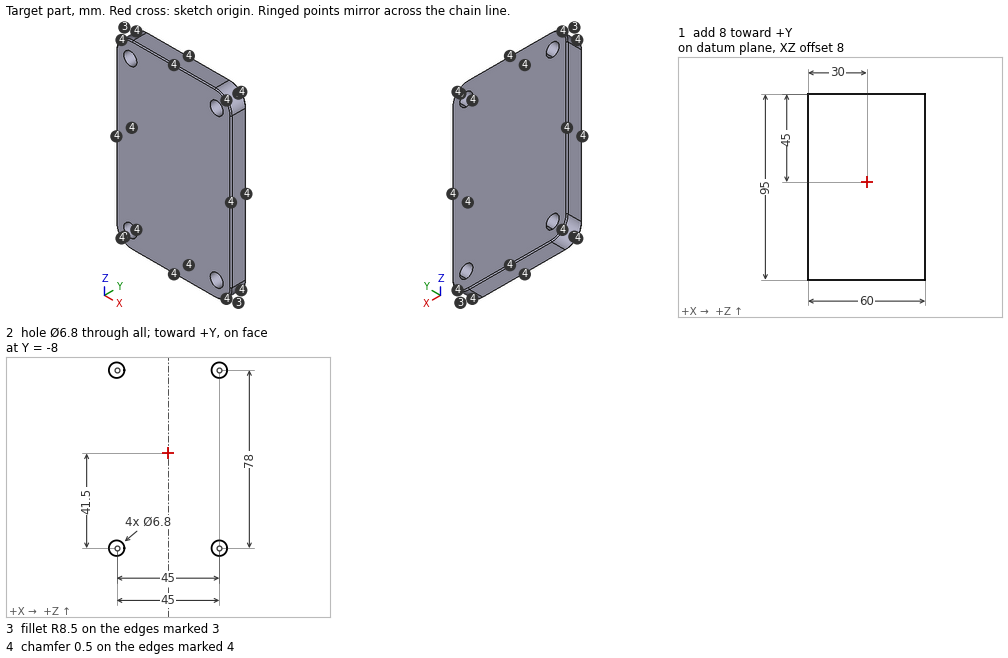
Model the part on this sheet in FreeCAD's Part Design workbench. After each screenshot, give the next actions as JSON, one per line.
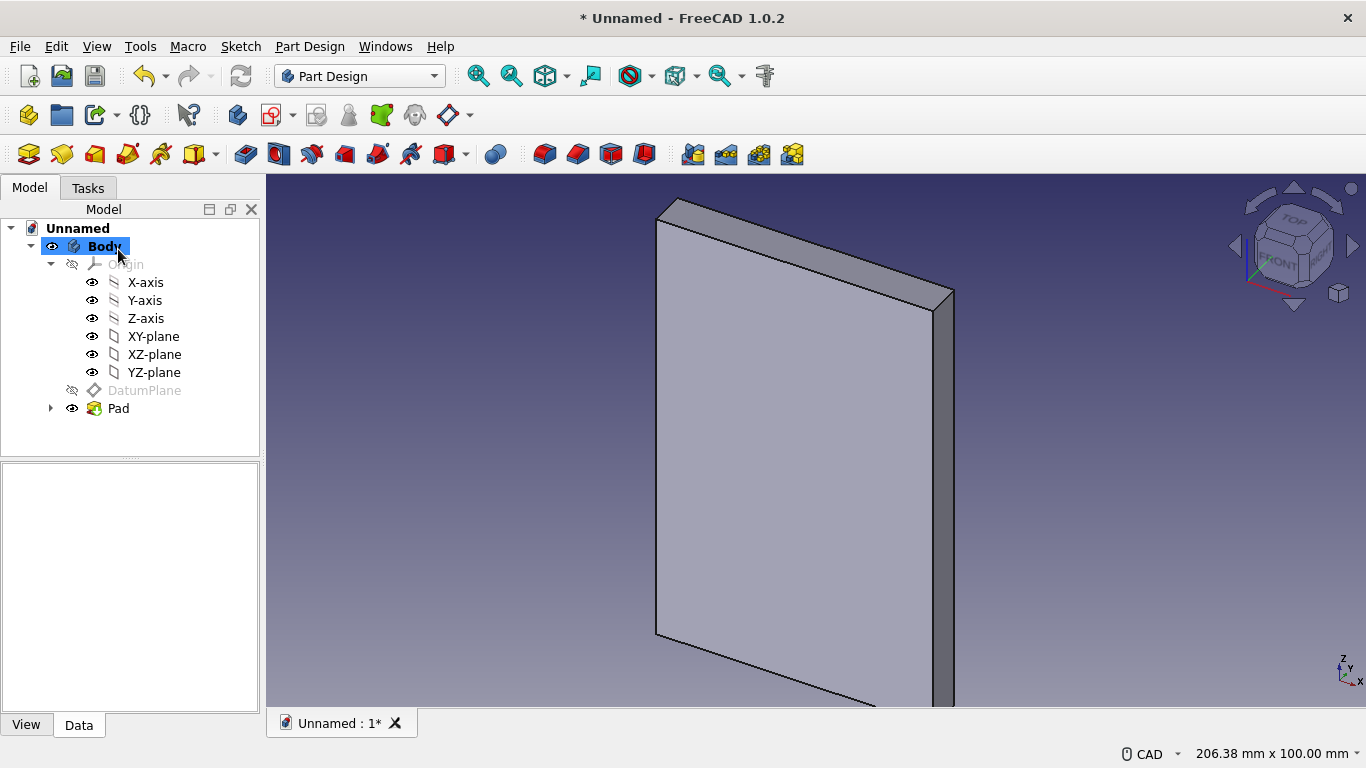
{"action": "left_click", "coordinate": [479, 76]}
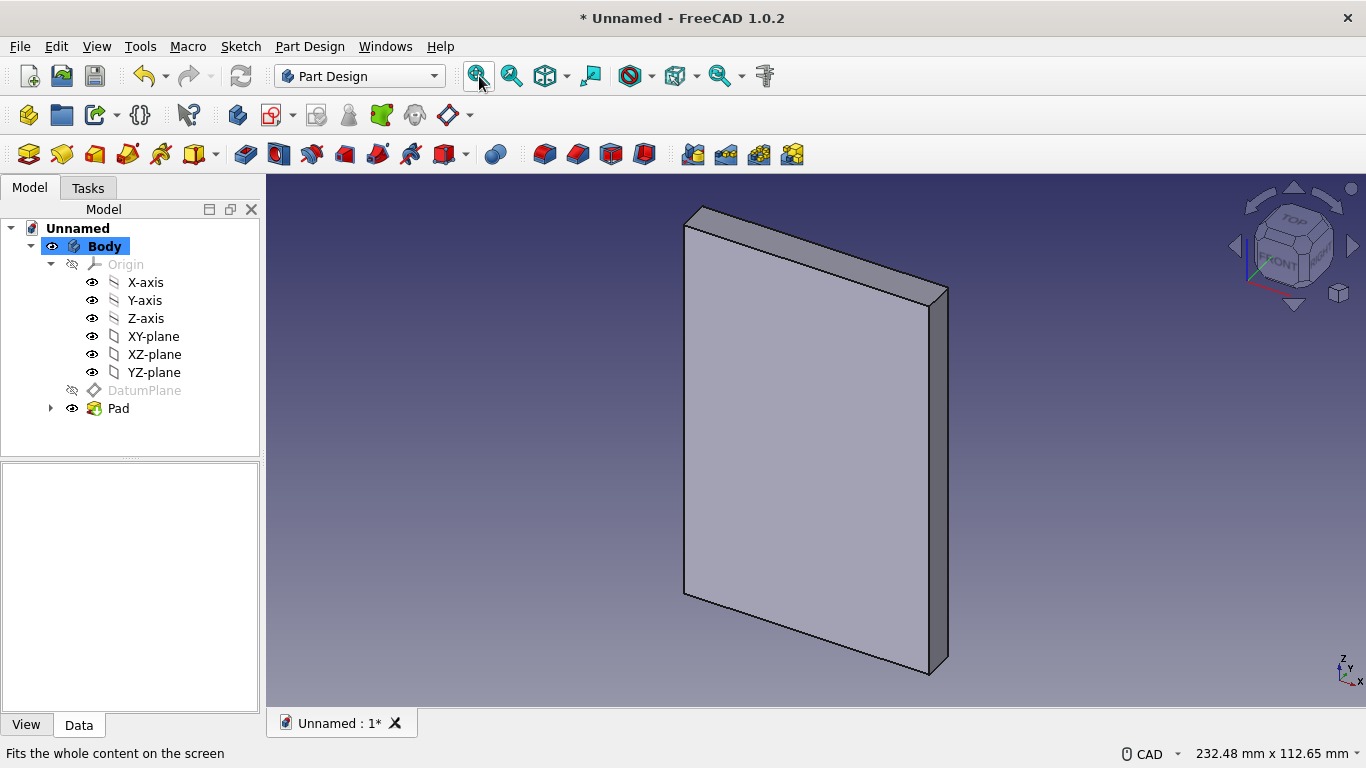
{"action": "left_click", "coordinate": [807, 396]}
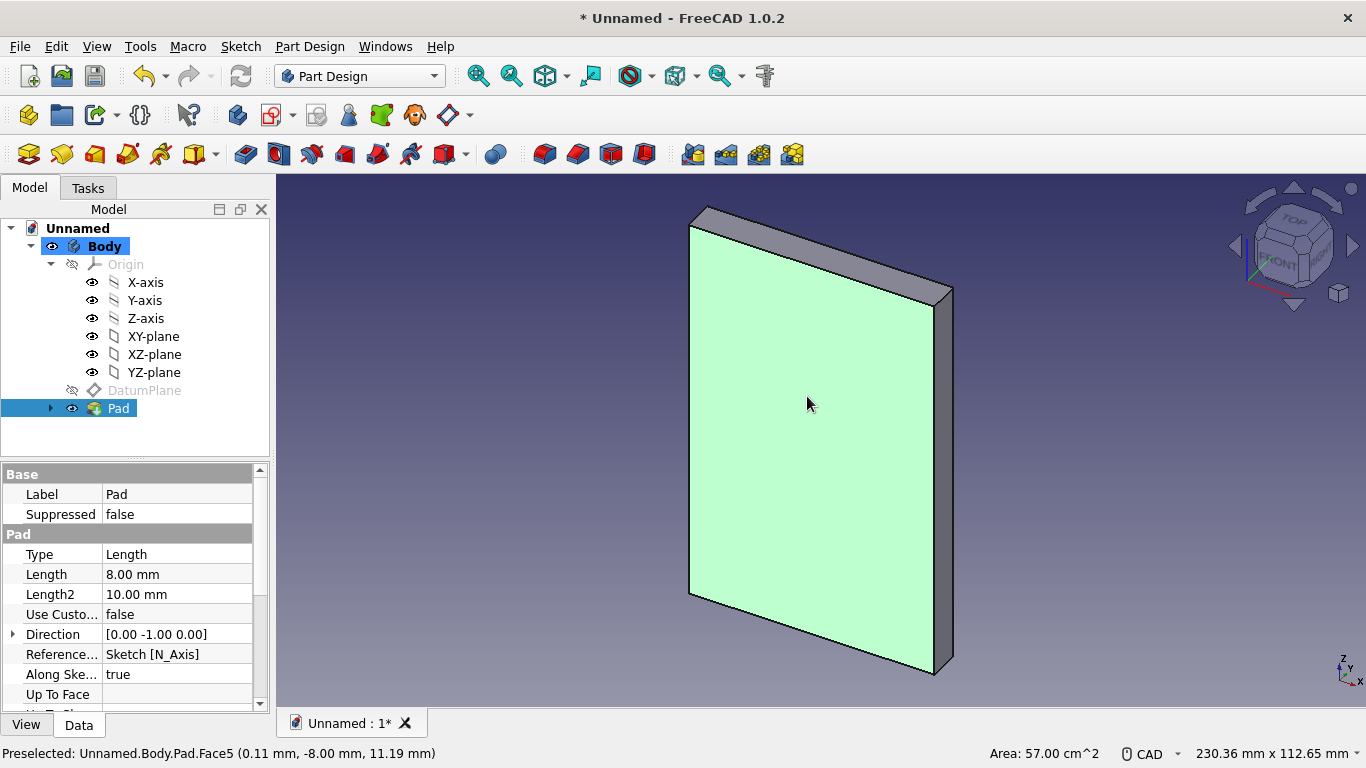
{"action": "left_click", "coordinate": [270, 116]}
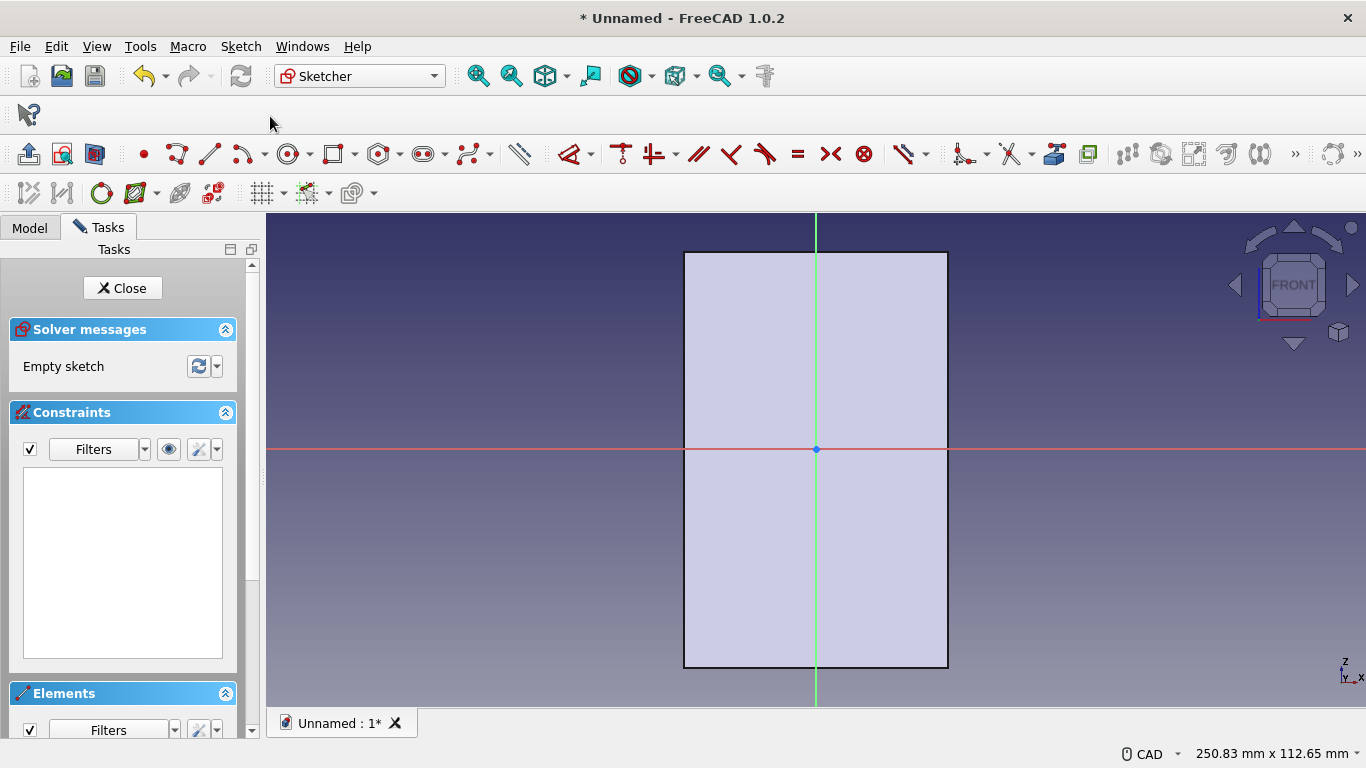
{"action": "left_click", "coordinate": [288, 154]}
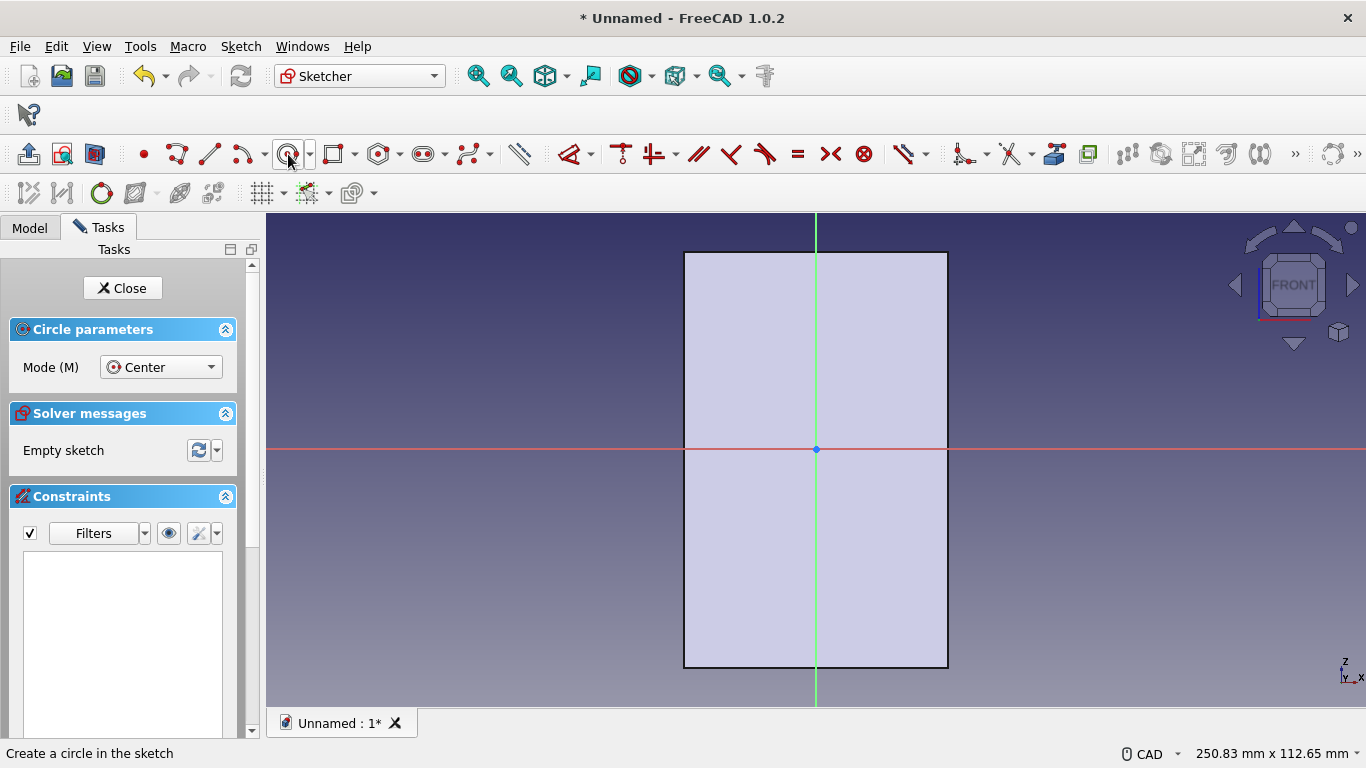
{"action": "scroll", "coordinate": [717, 631], "scroll_direction": "up", "scroll_amount": 3}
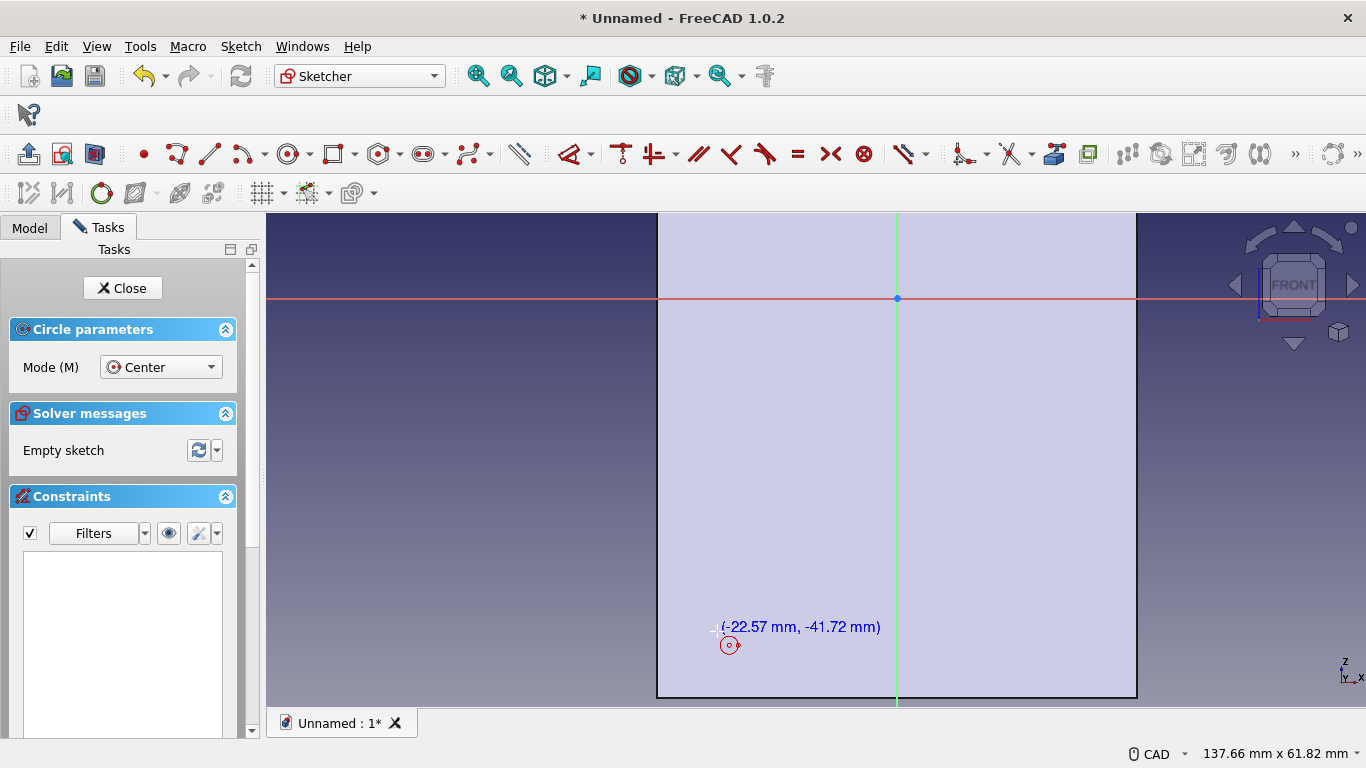
{"action": "left_click", "coordinate": [717, 630]}
{"action": "left_click", "coordinate": [736, 611]}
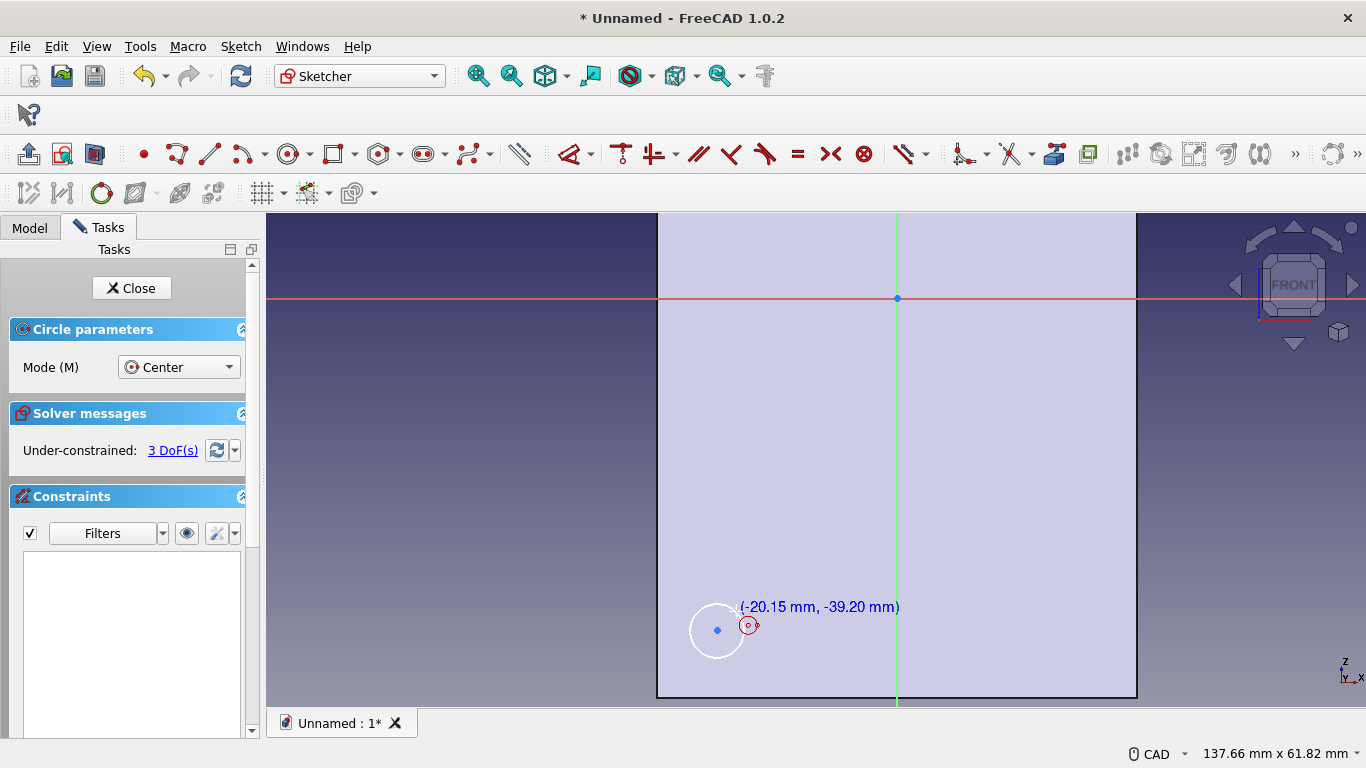
{"action": "left_click", "coordinate": [1077, 630]}
{"action": "left_click", "coordinate": [1096, 611]}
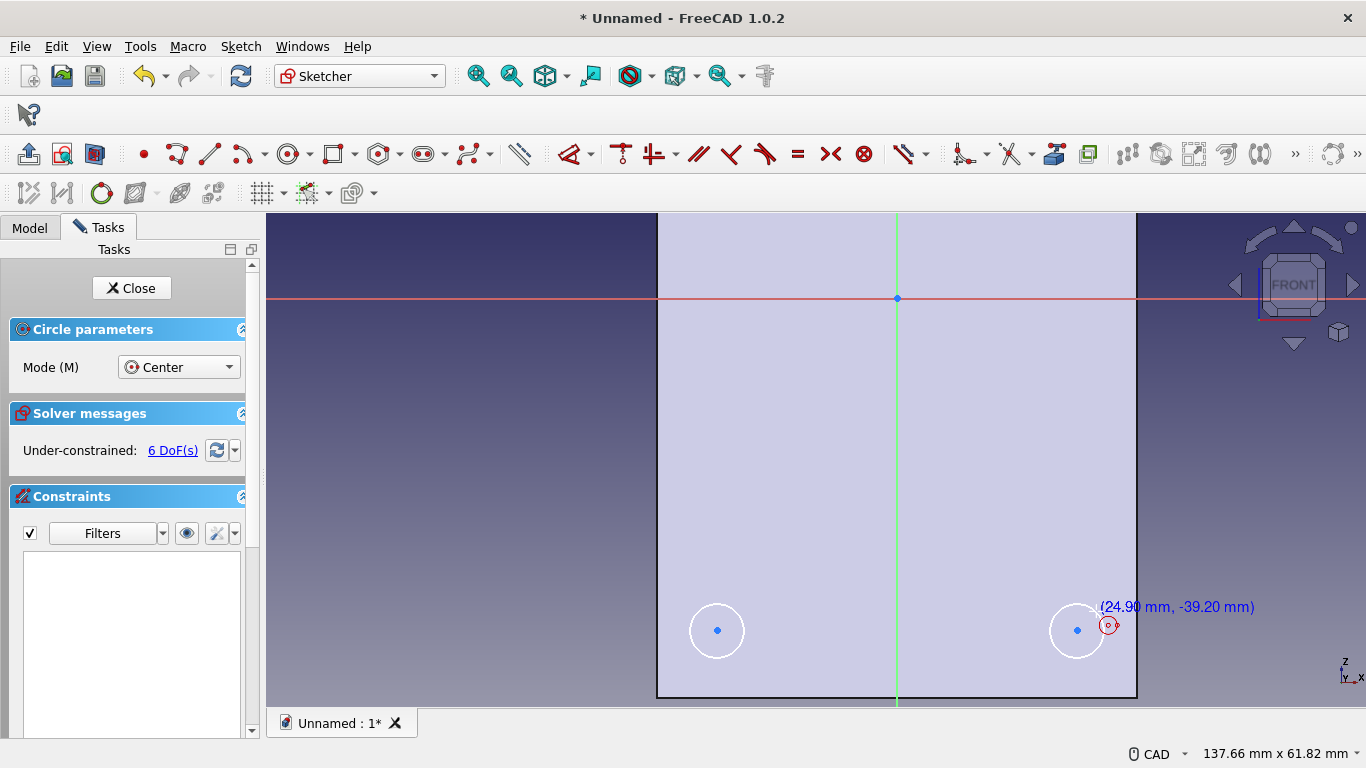
{"action": "scroll", "coordinate": [625, 575], "scroll_direction": "down", "scroll_amount": 4}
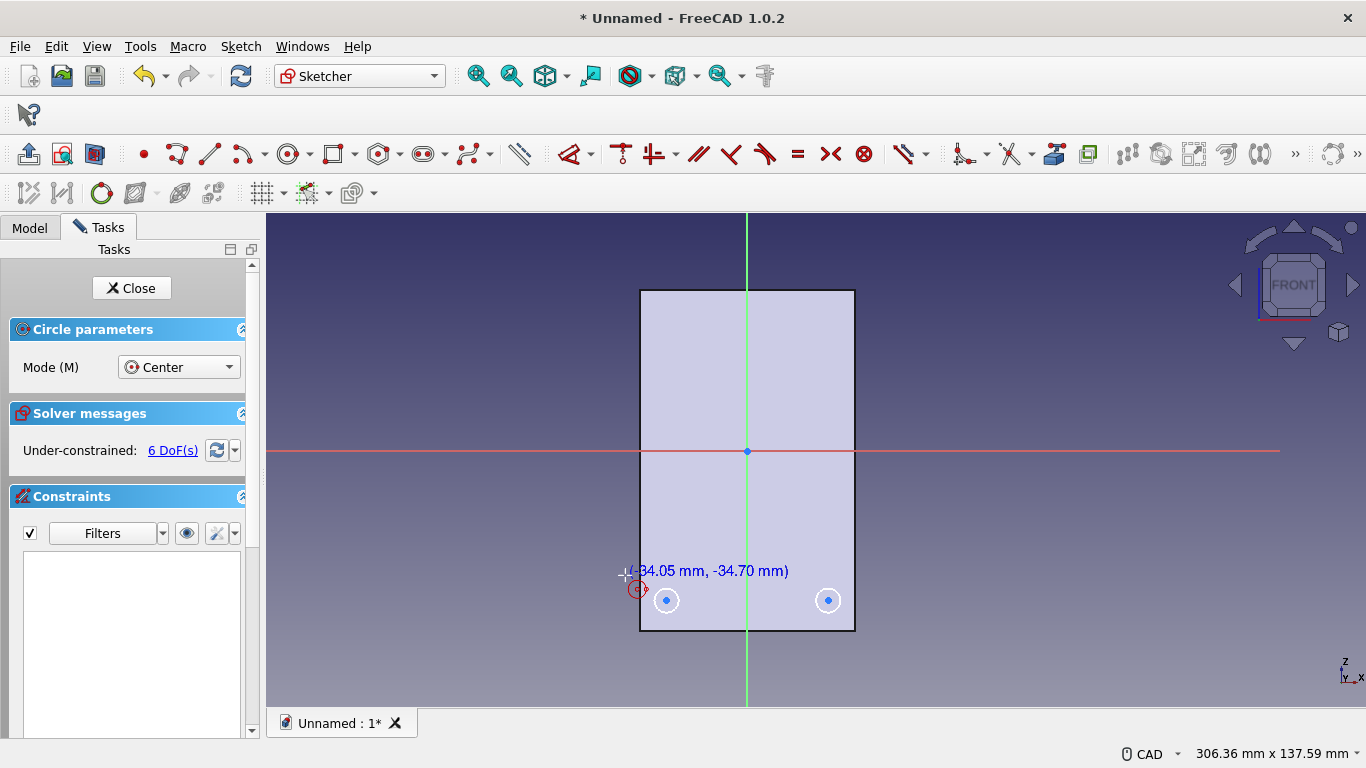
{"action": "scroll", "coordinate": [828, 320], "scroll_direction": "up", "scroll_amount": 4}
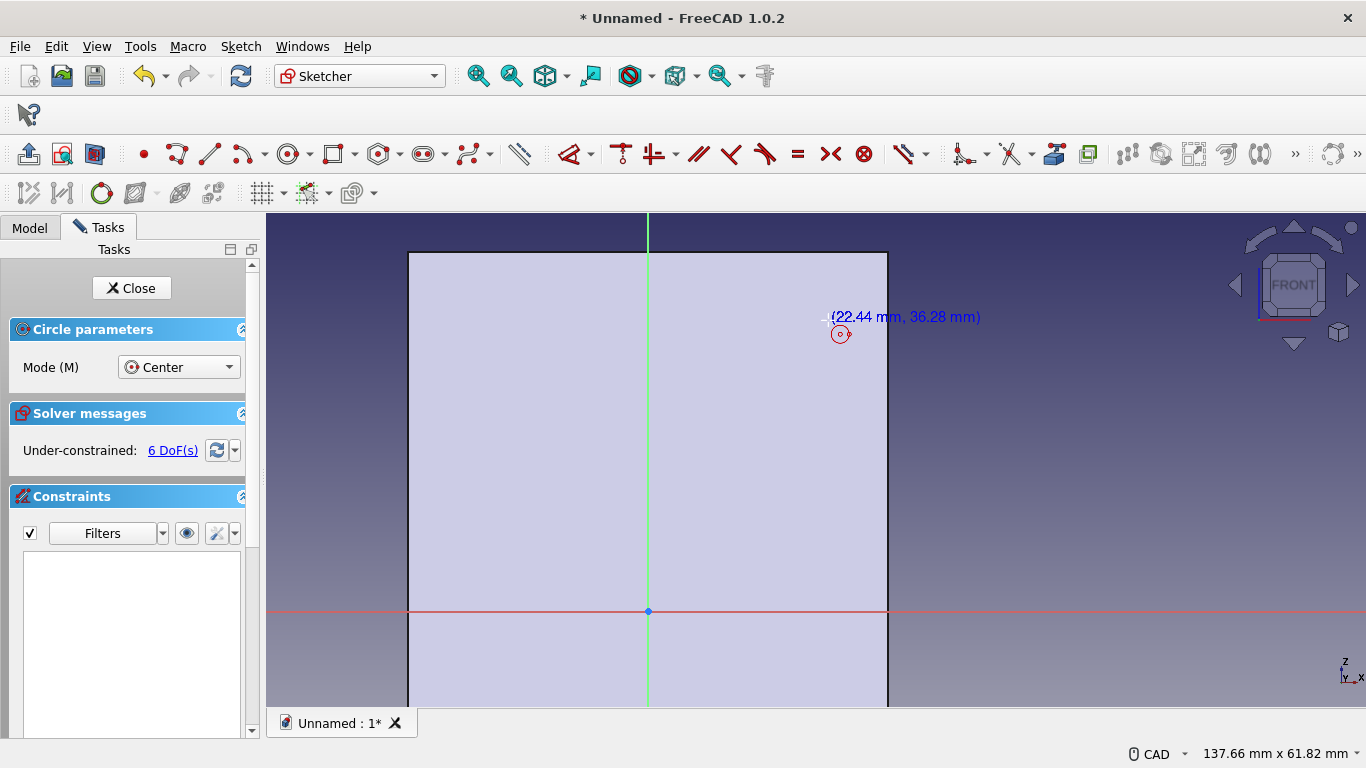
{"action": "left_click", "coordinate": [828, 320]}
{"action": "left_click", "coordinate": [847, 301]}